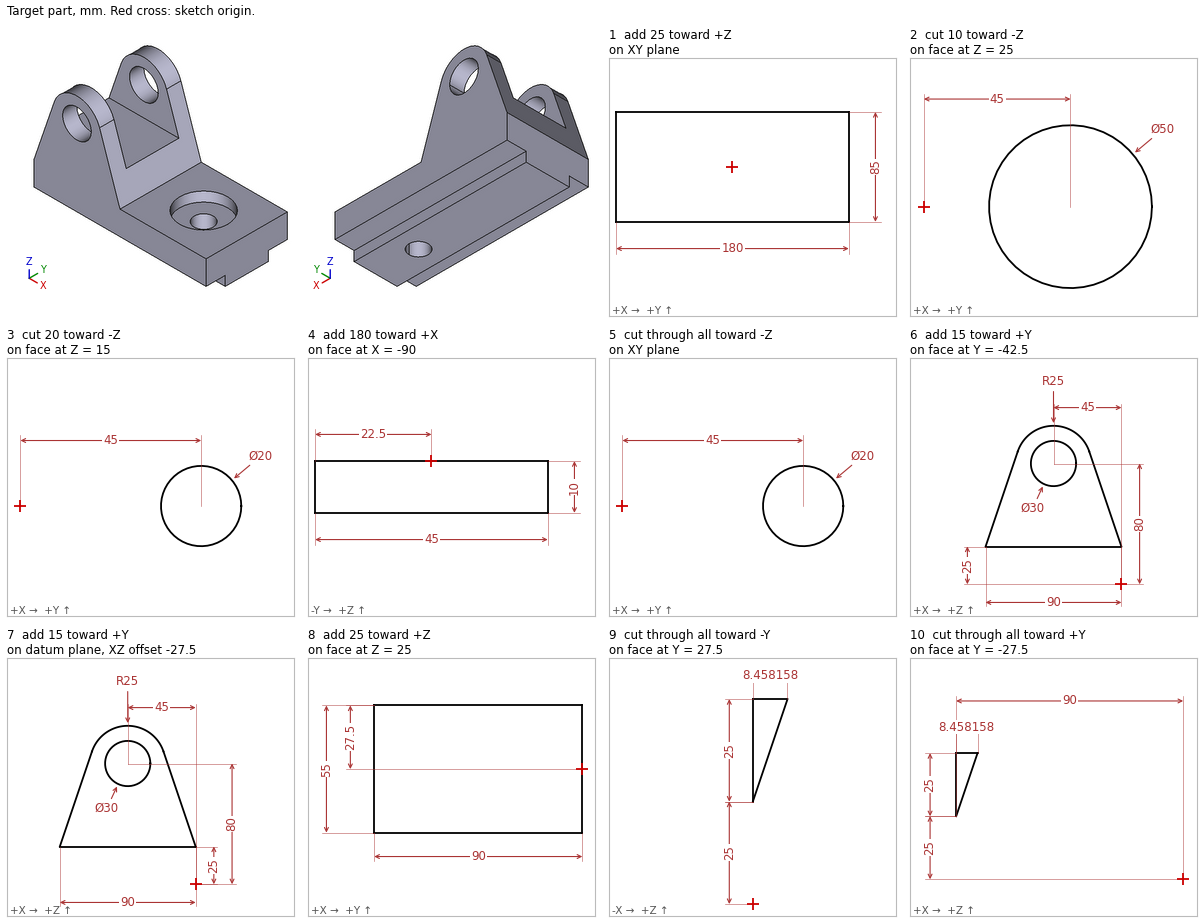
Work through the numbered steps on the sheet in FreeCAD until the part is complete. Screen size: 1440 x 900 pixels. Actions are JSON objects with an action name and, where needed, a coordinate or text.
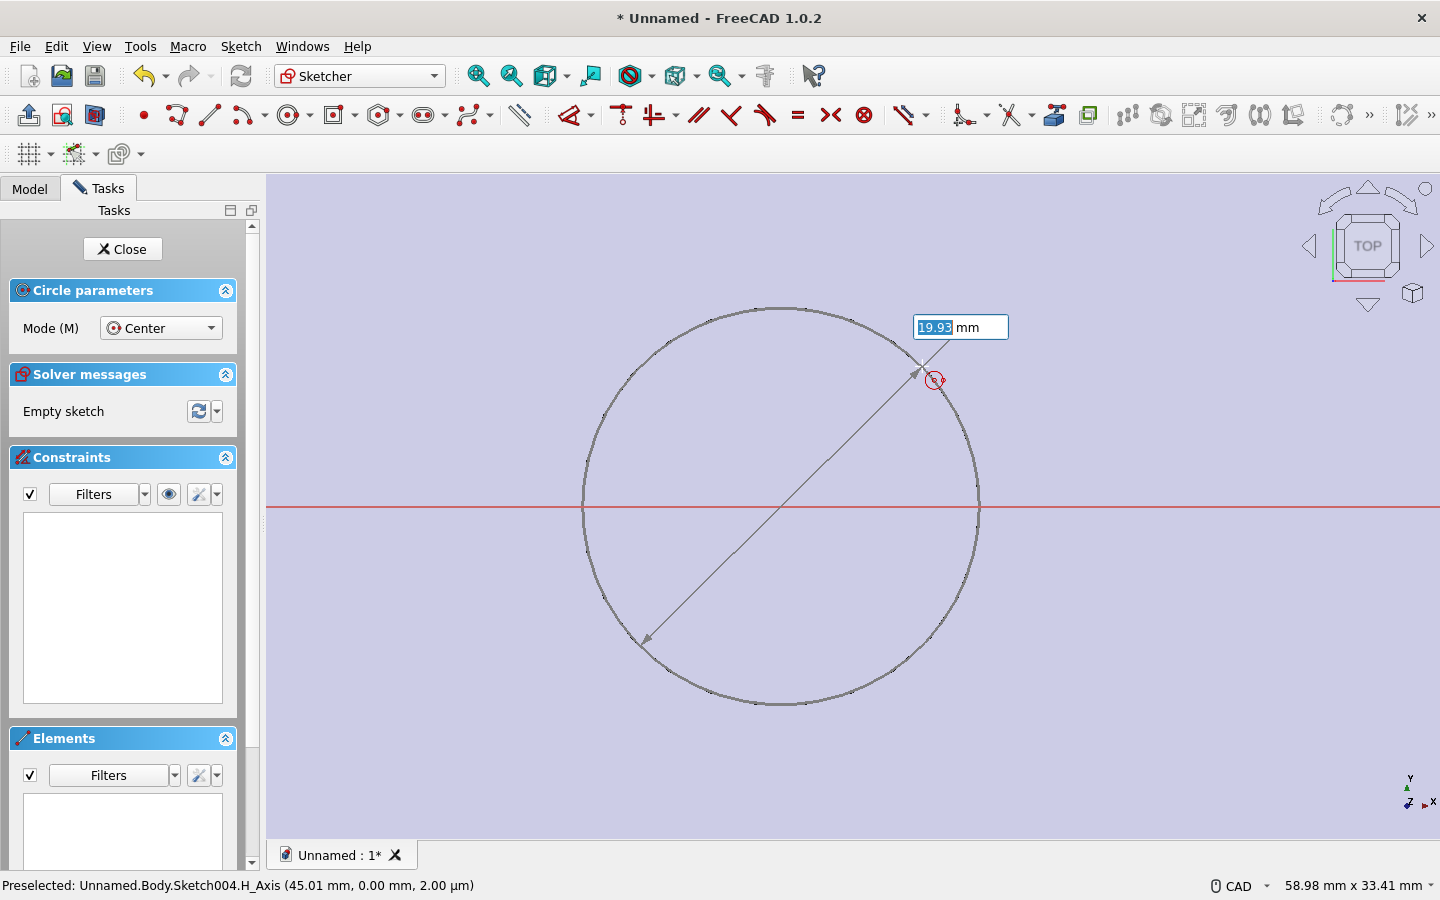
{"action": "type", "text": "20"}
{"action": "key", "text": "Return"}
{"action": "key", "text": "Escape"}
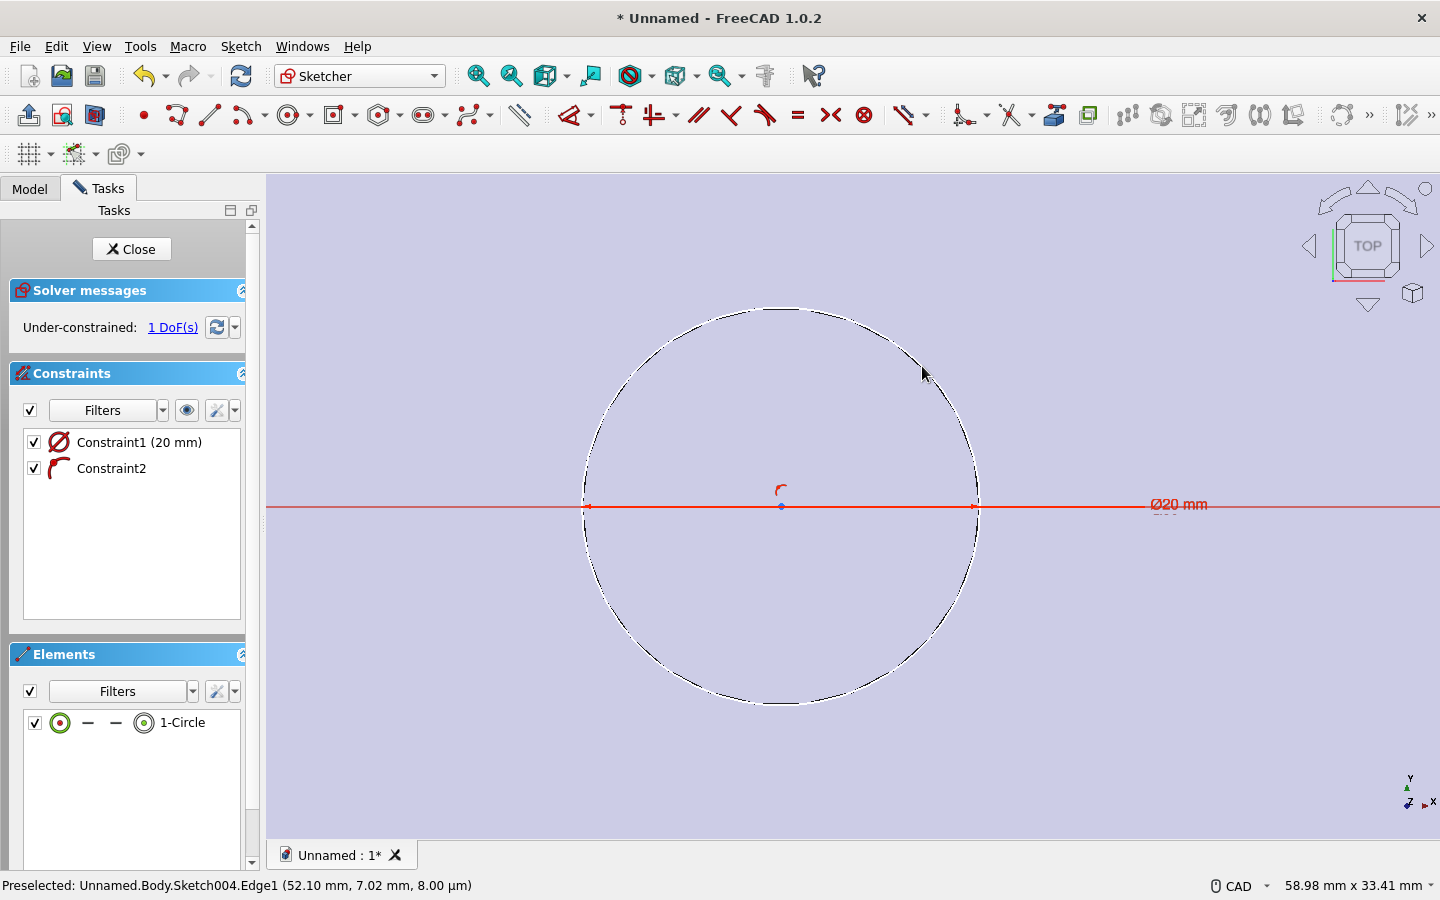
{"action": "left_click", "coordinate": [568, 116]}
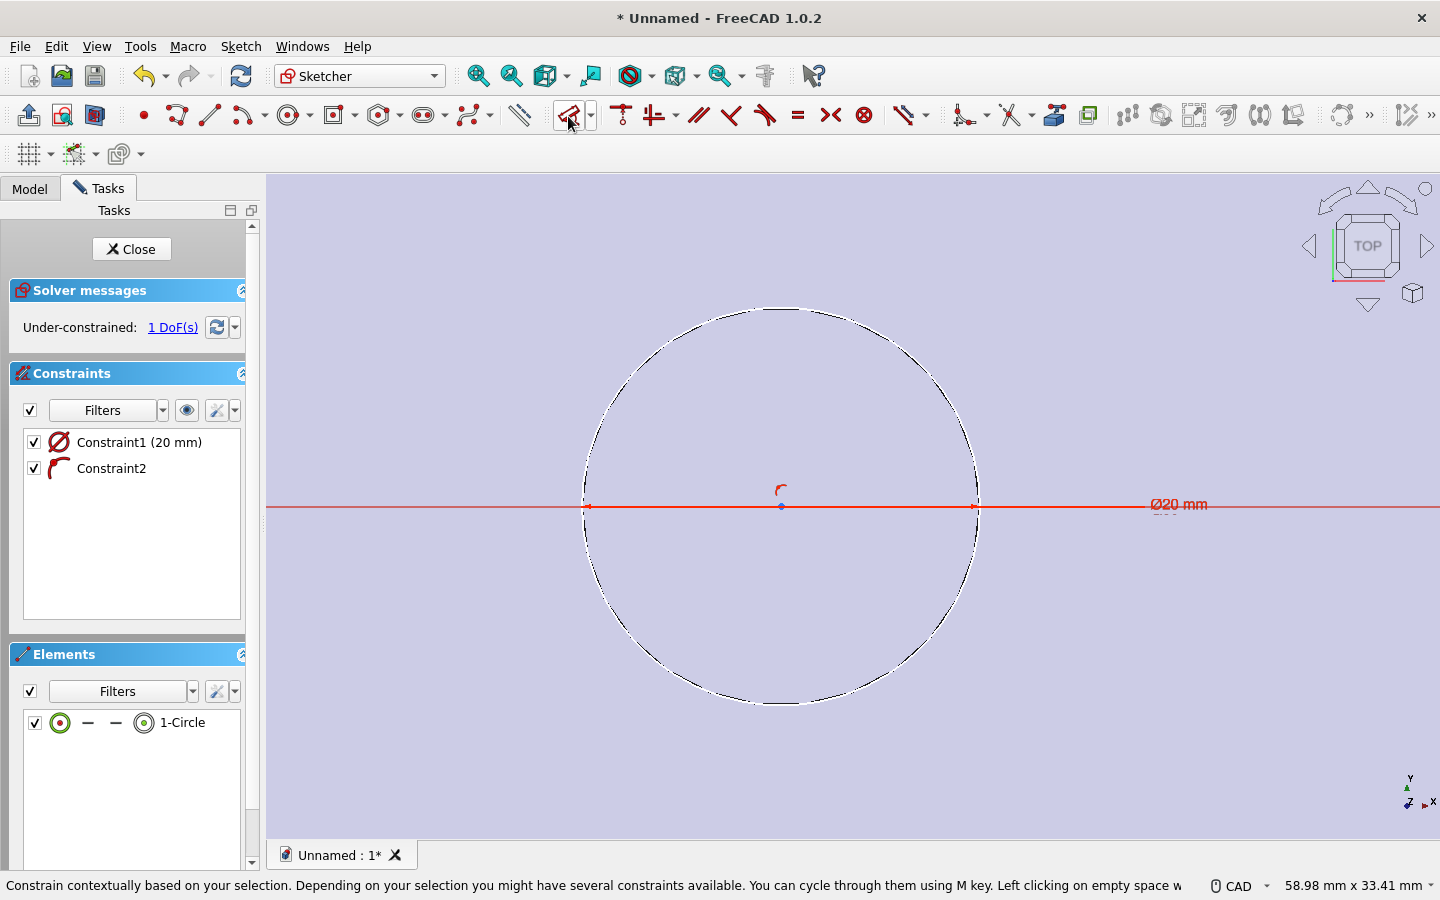
{"action": "left_click", "coordinate": [781, 506]}
{"action": "left_click", "coordinate": [537, 540]}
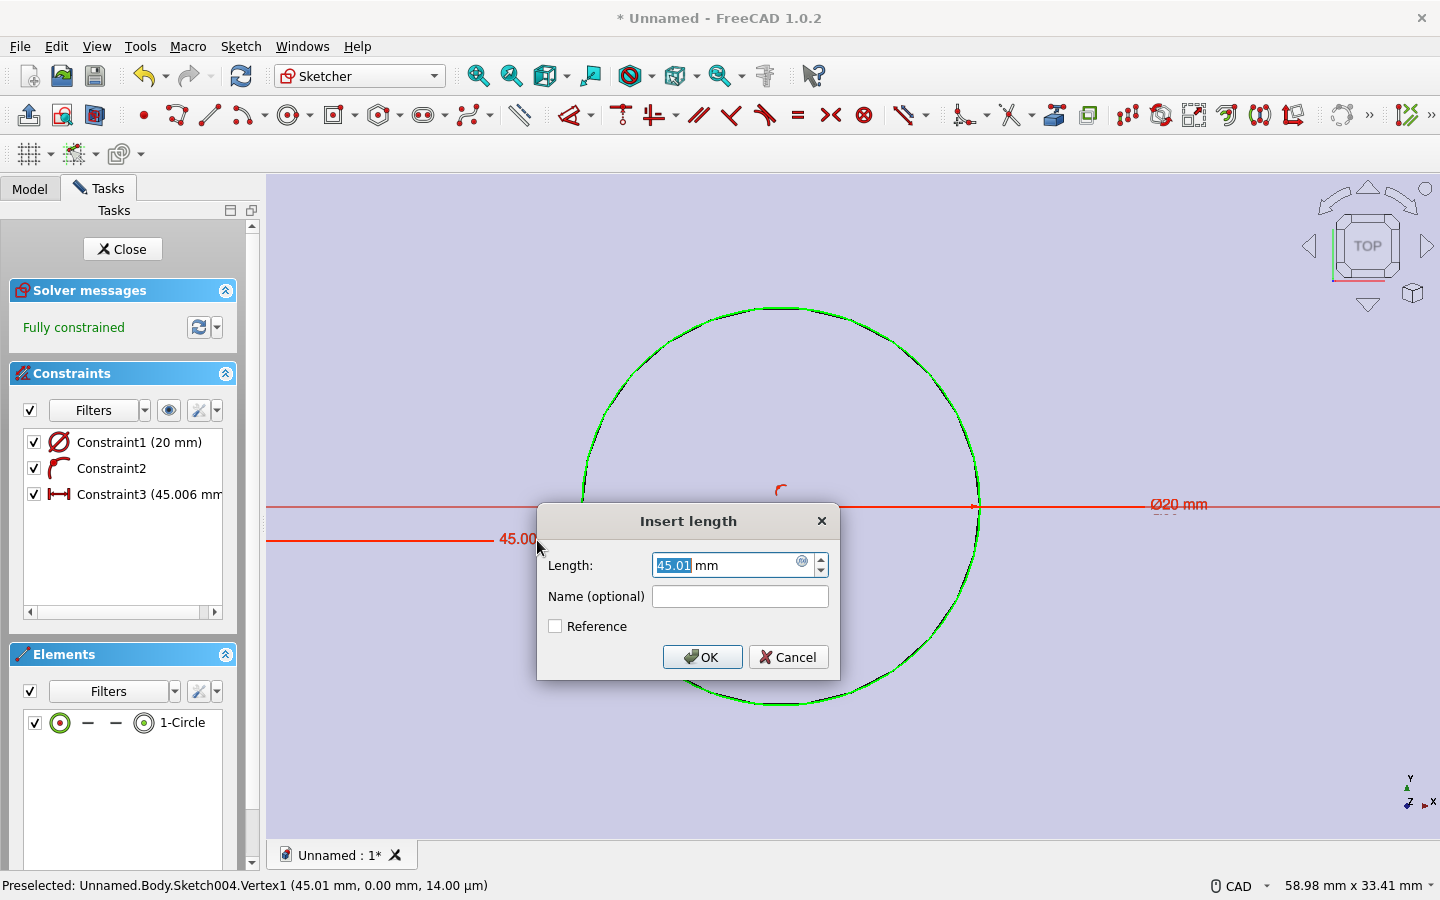
{"action": "type", "text": "45"}
{"action": "key", "text": "Return"}
{"action": "key", "text": "Escape"}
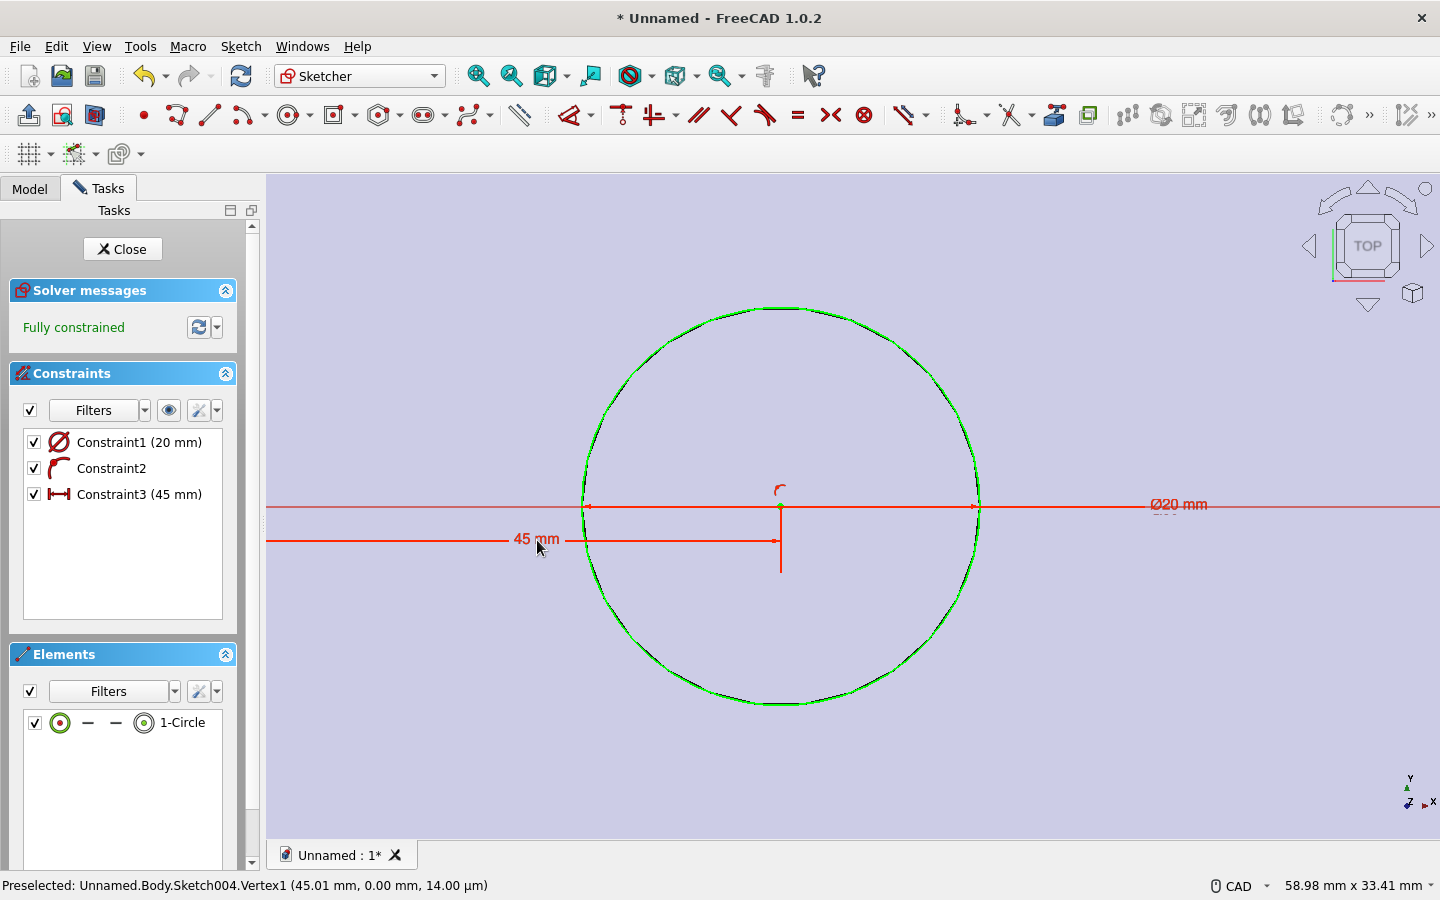
{"action": "left_click", "coordinate": [123, 249]}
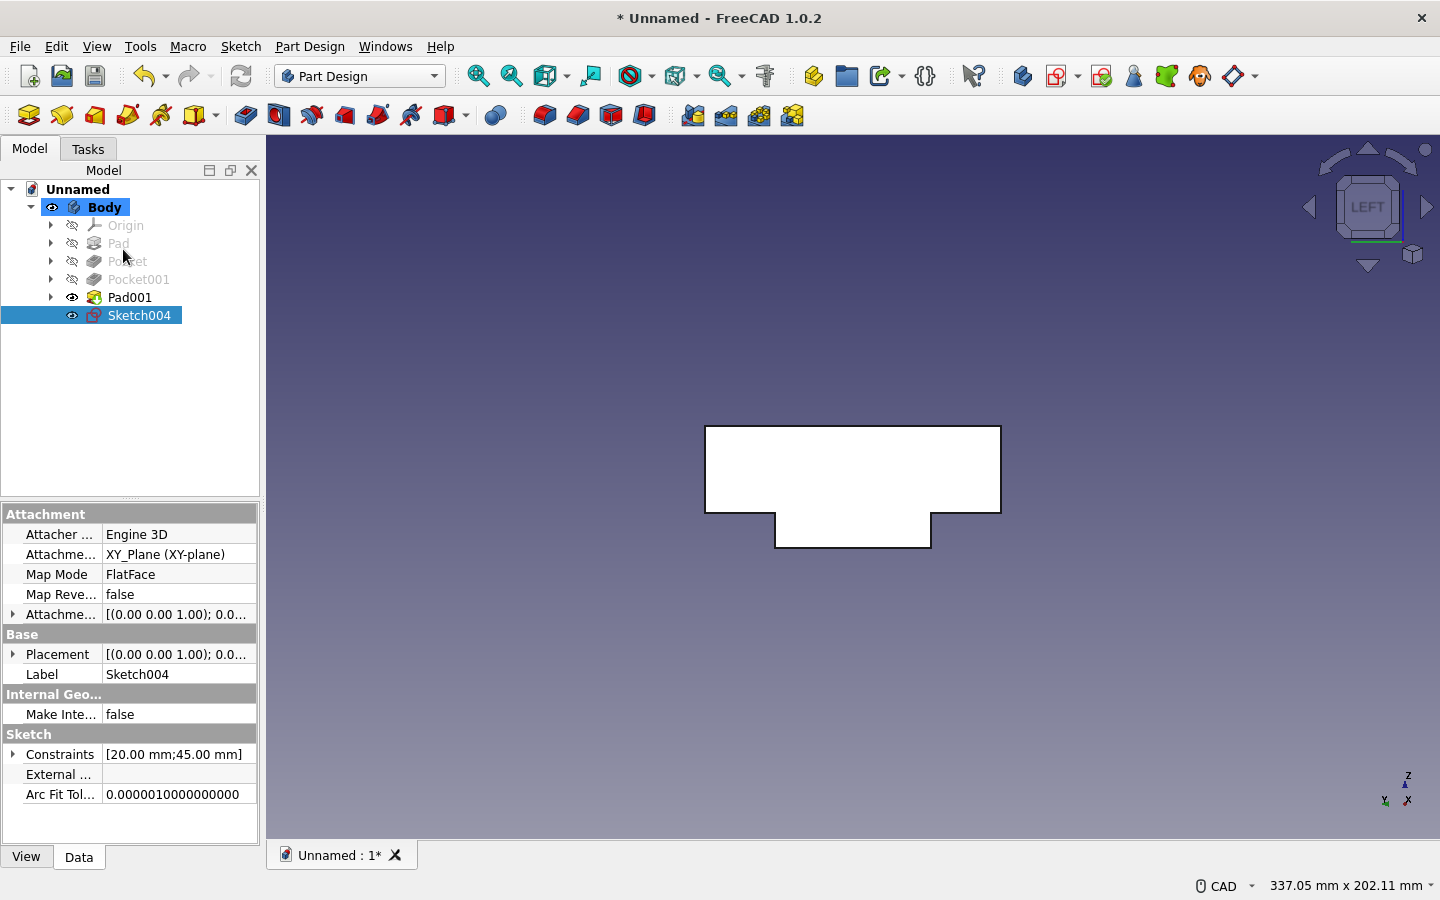
{"action": "left_click", "coordinate": [246, 116]}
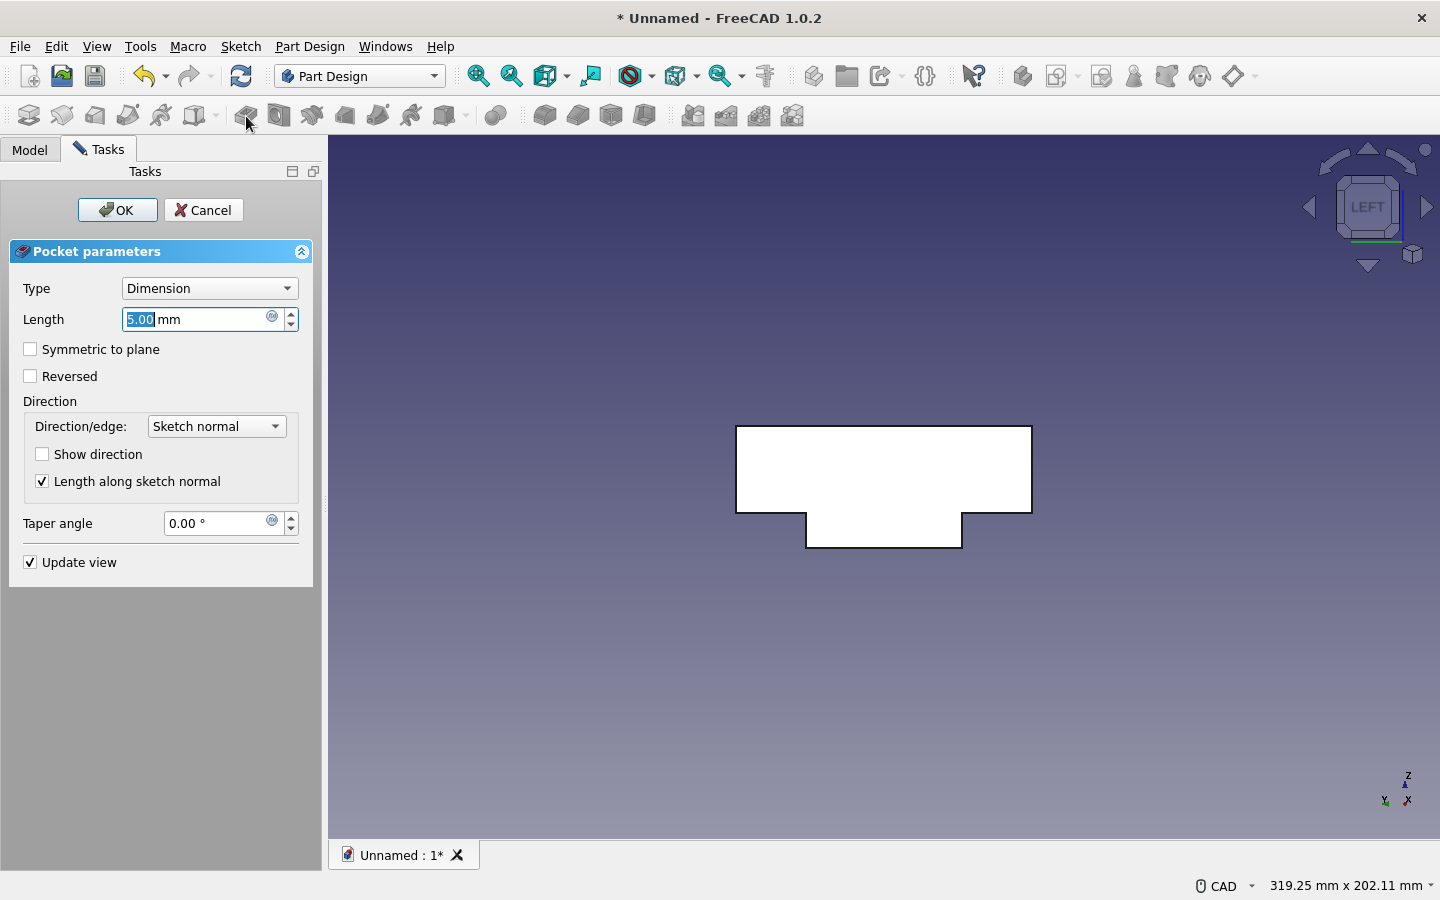
{"action": "left_click", "coordinate": [210, 288]}